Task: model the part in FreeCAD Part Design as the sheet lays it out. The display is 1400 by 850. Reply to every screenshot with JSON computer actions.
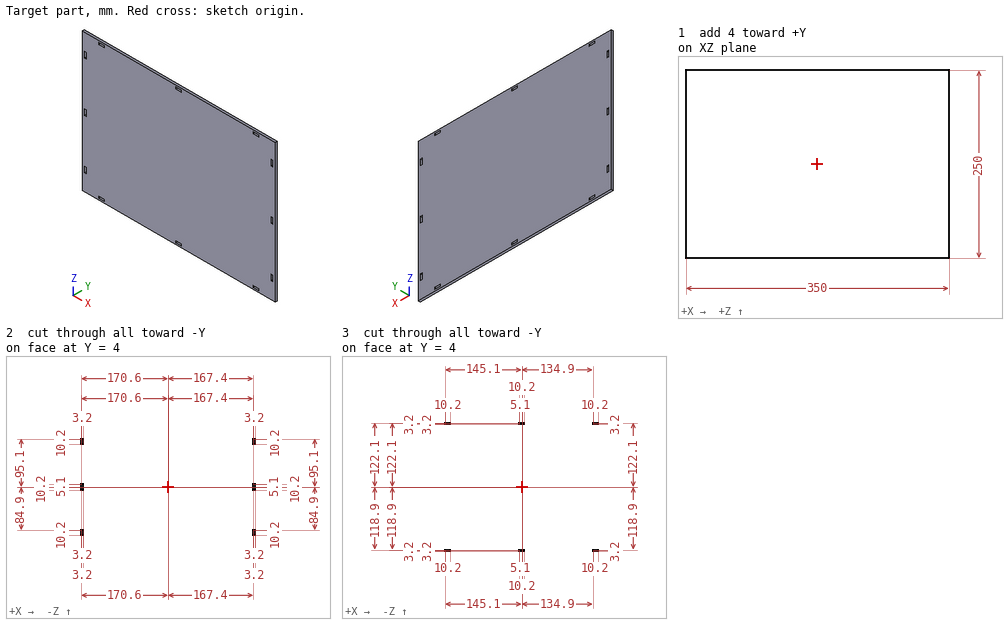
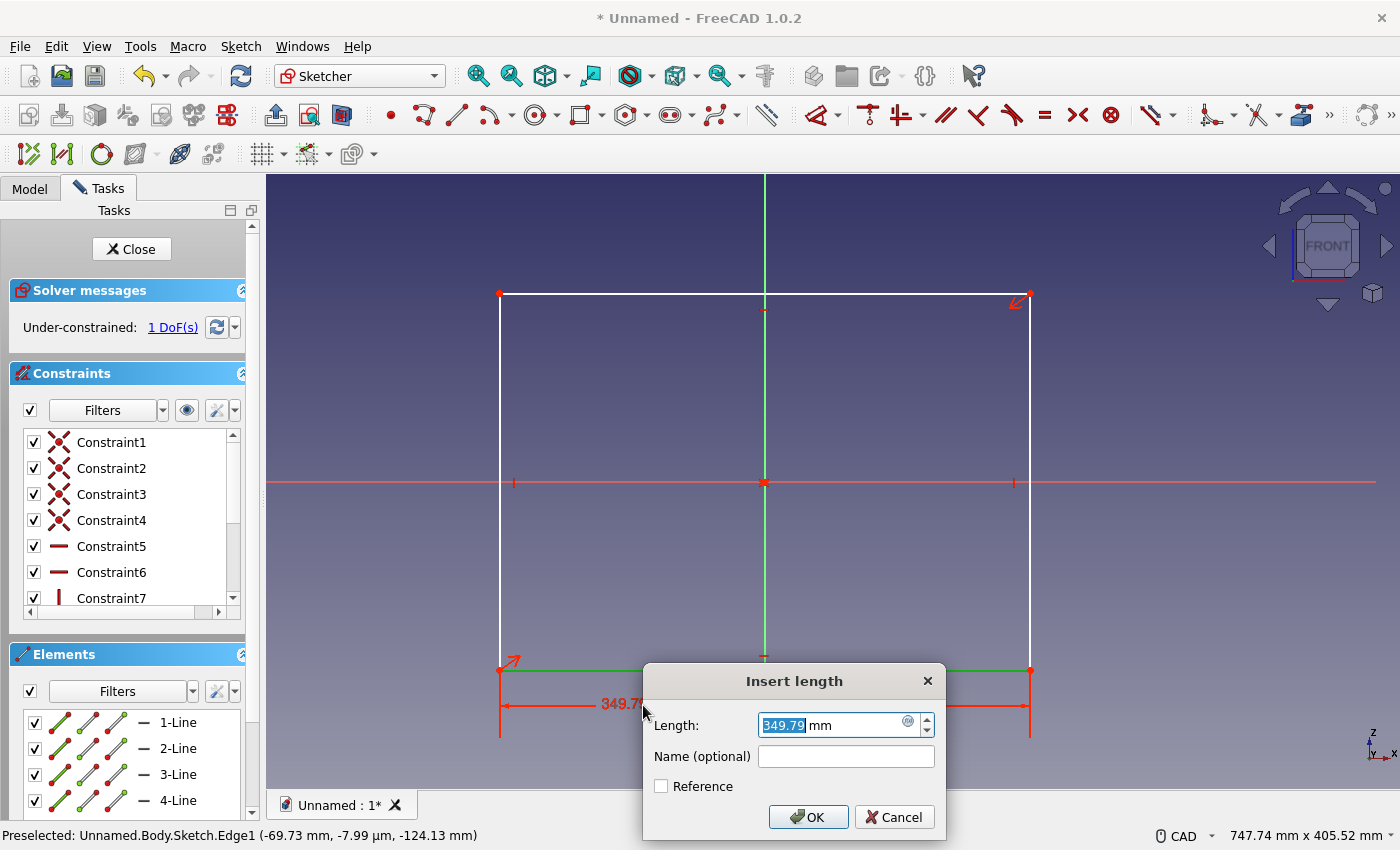
{"action": "type", "text": "350"}
{"action": "key", "text": "Return"}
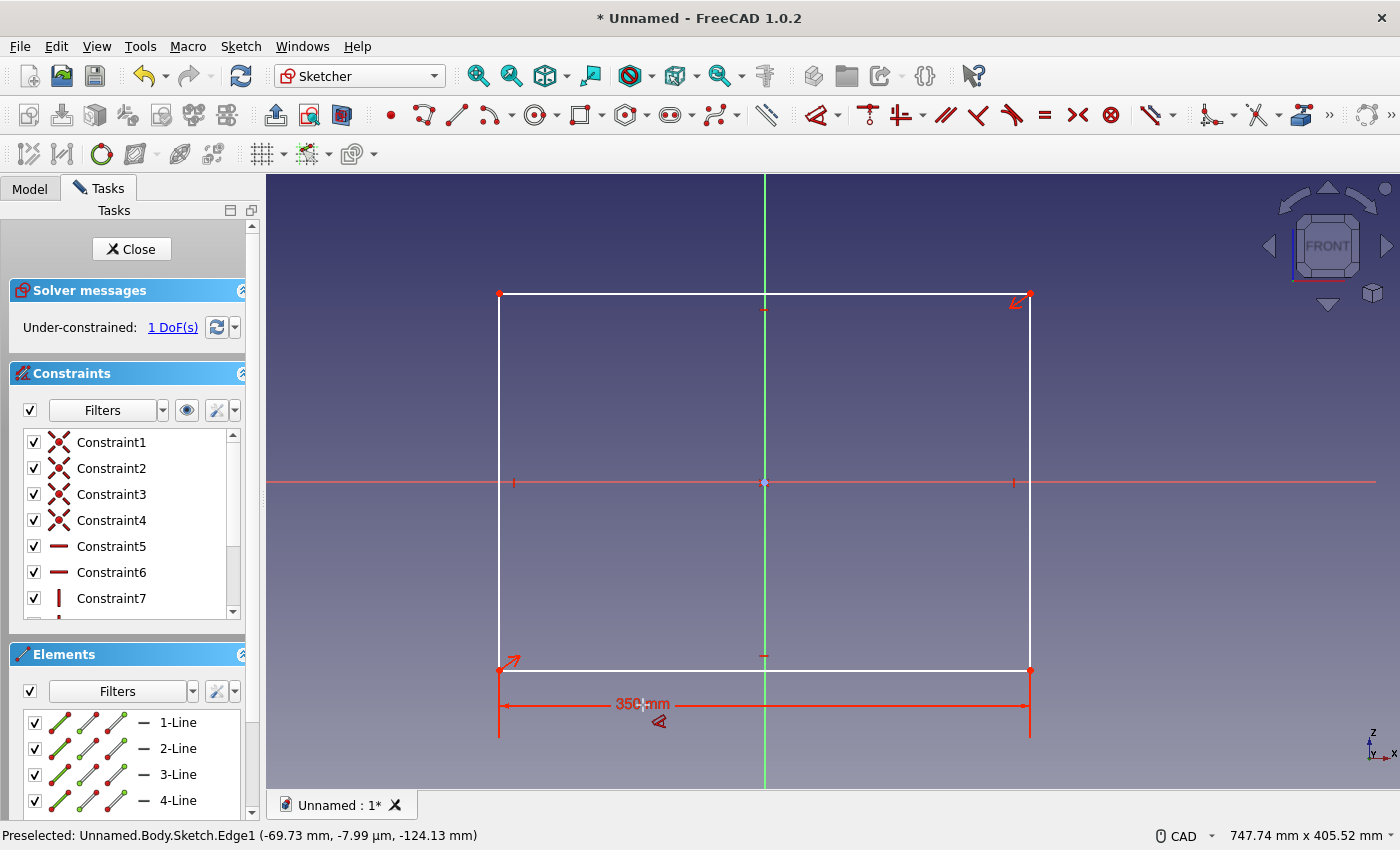
{"action": "left_click", "coordinate": [1030, 558]}
{"action": "left_click", "coordinate": [1064, 396]}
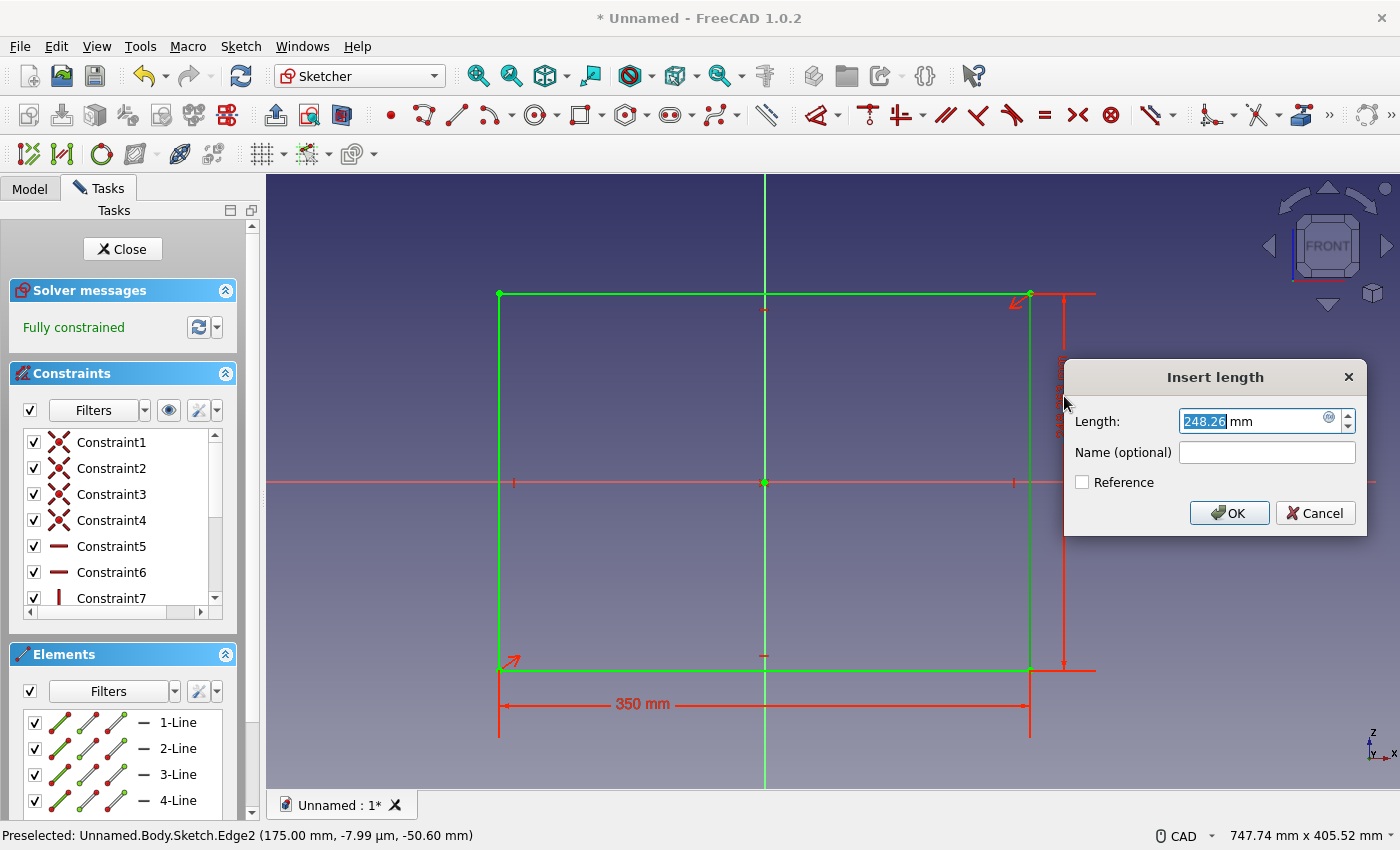
{"action": "type", "text": "250"}
{"action": "key", "text": "Return"}
{"action": "key", "text": "Escape"}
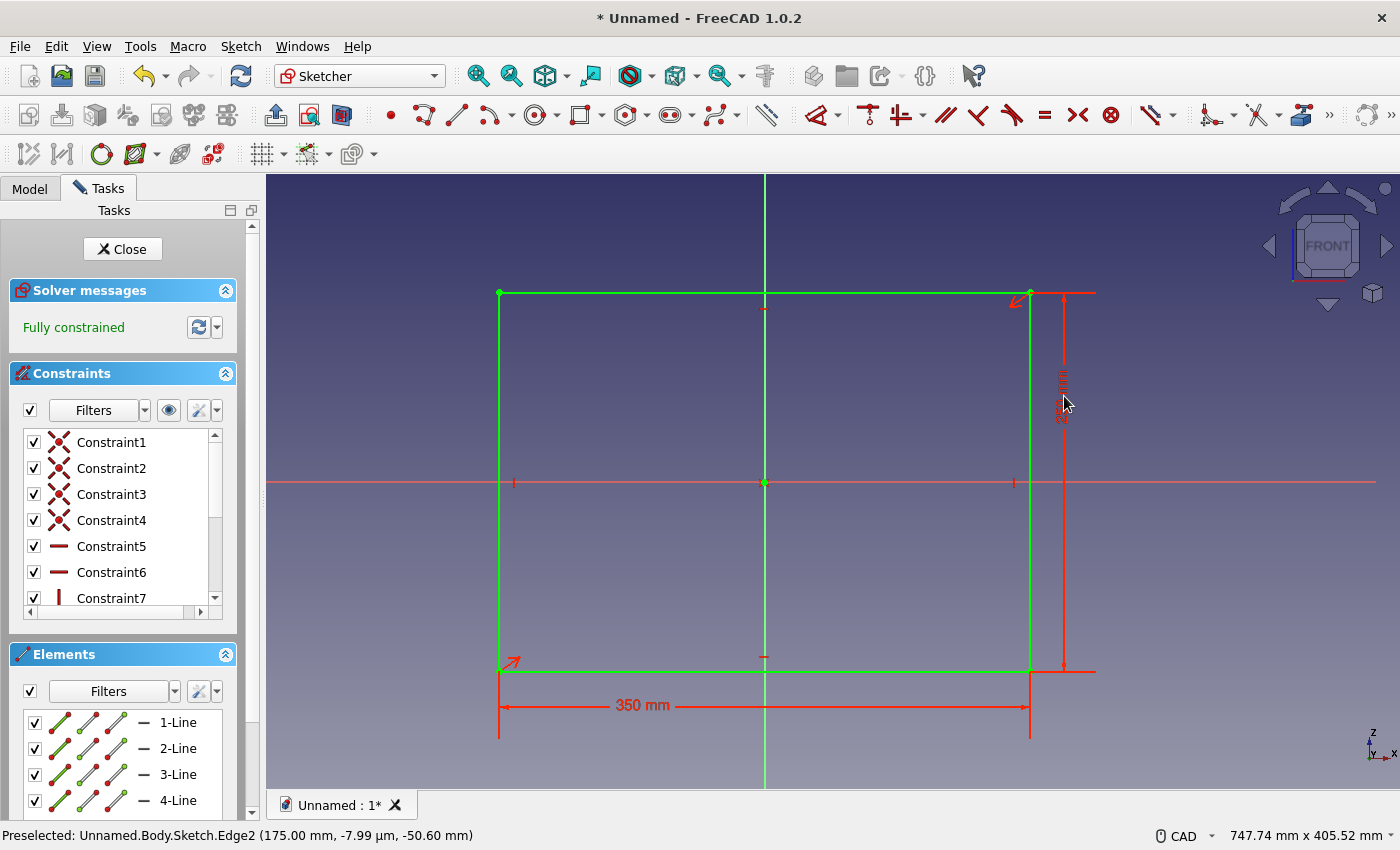
{"action": "left_click", "coordinate": [123, 249]}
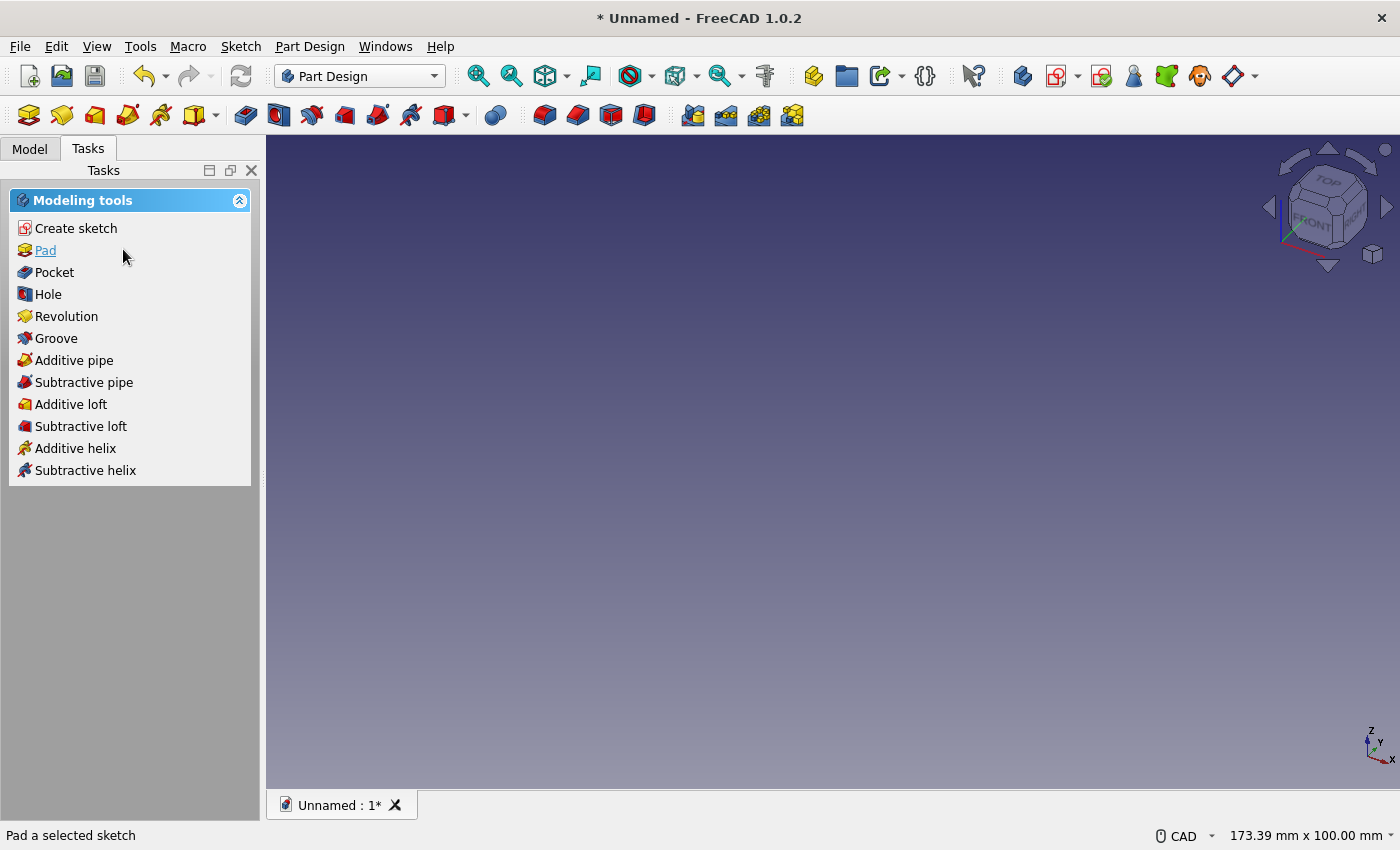
{"action": "left_click", "coordinate": [29, 116]}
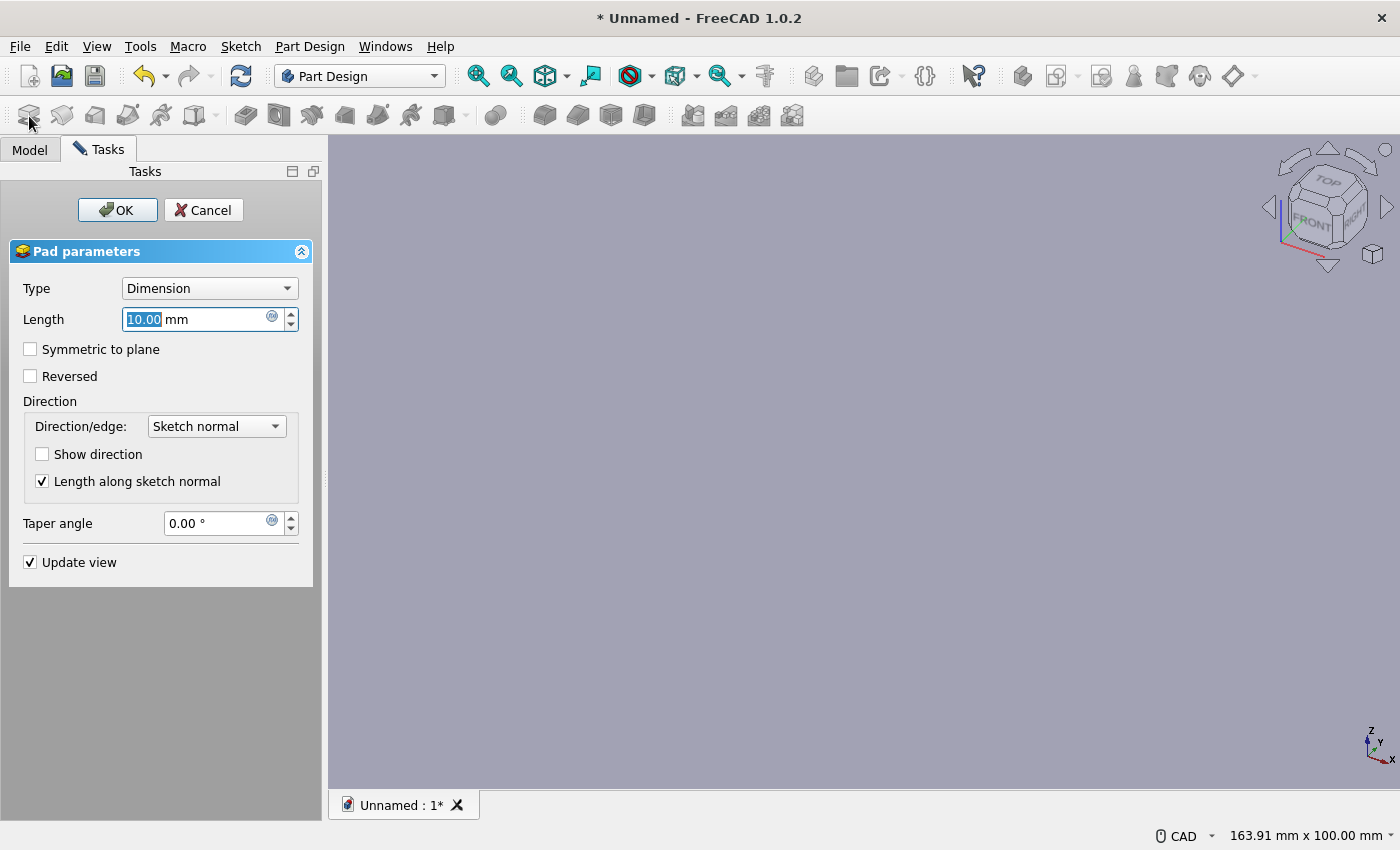
{"action": "type", "text": "4"}
{"action": "key", "text": "Tab"}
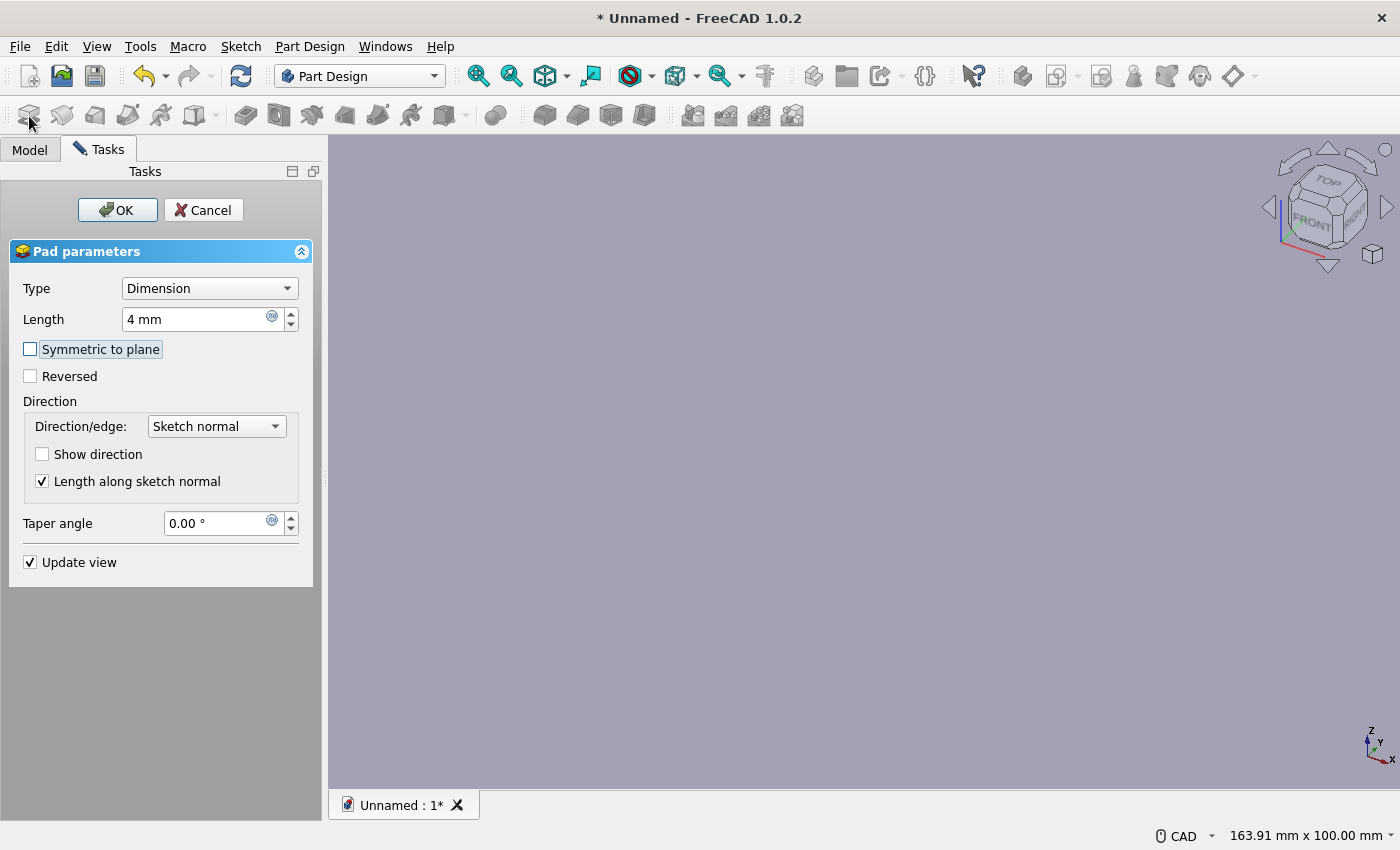
{"action": "left_click", "coordinate": [31, 376]}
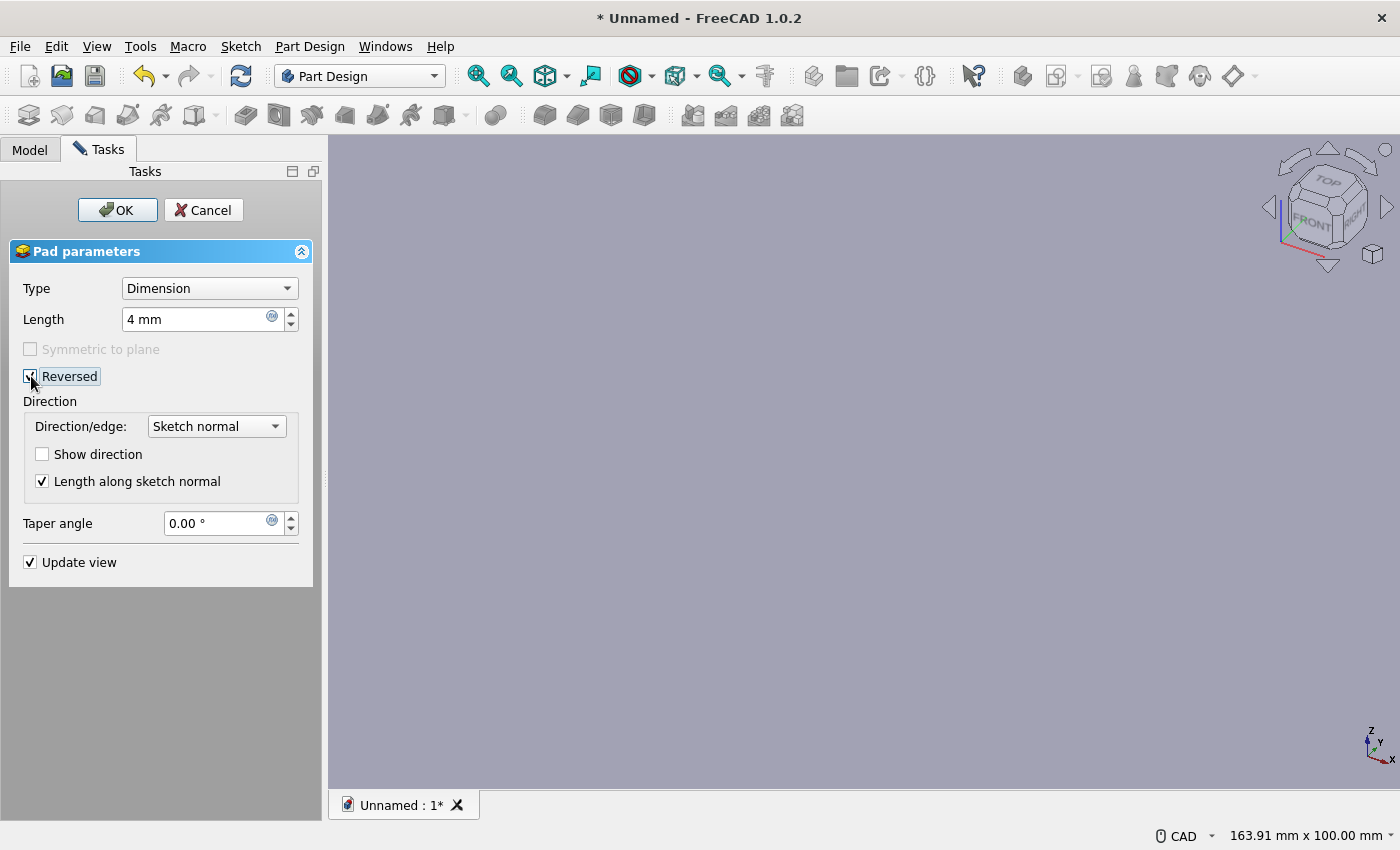
{"action": "left_click", "coordinate": [118, 210]}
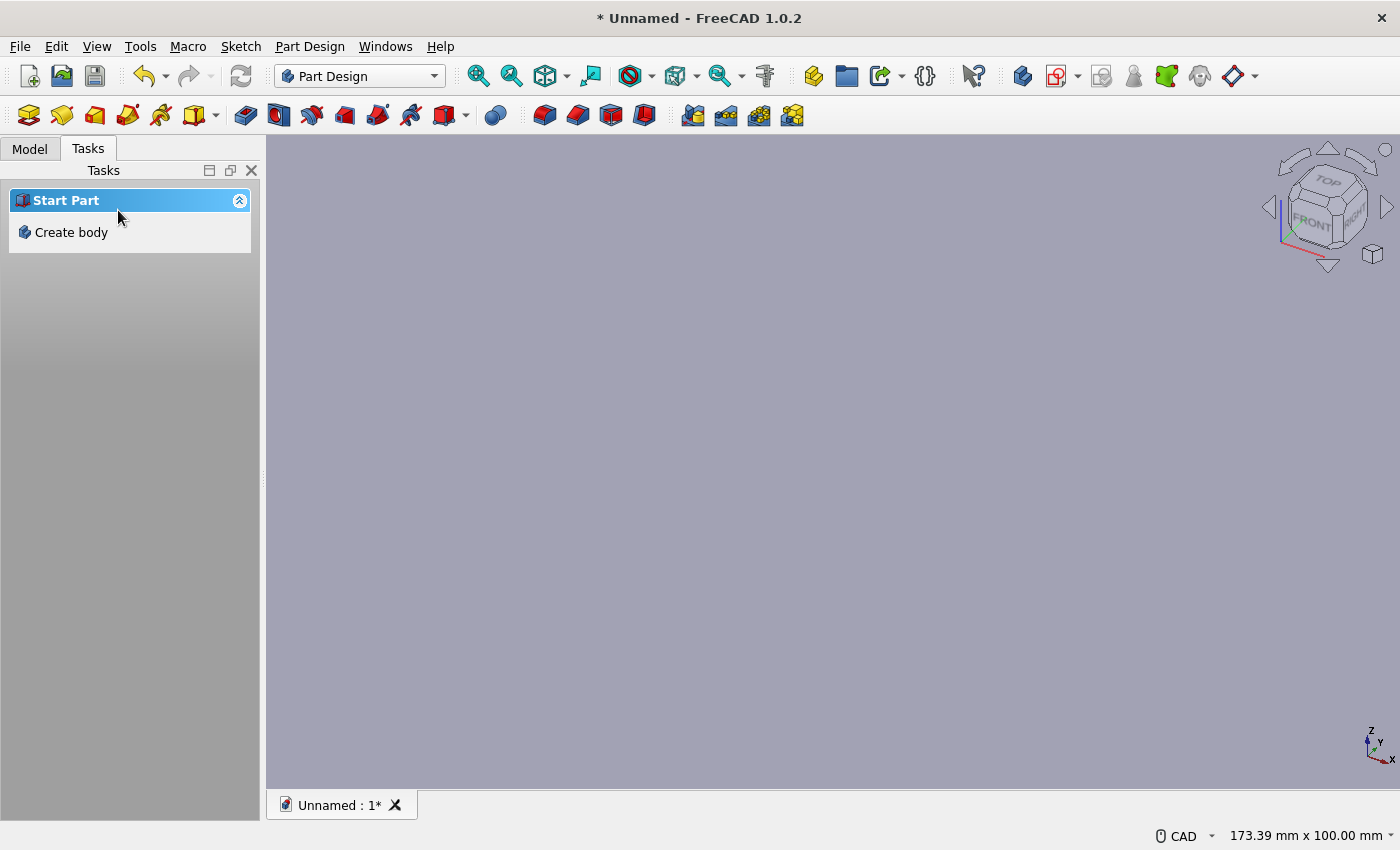
{"action": "left_click", "coordinate": [479, 76]}